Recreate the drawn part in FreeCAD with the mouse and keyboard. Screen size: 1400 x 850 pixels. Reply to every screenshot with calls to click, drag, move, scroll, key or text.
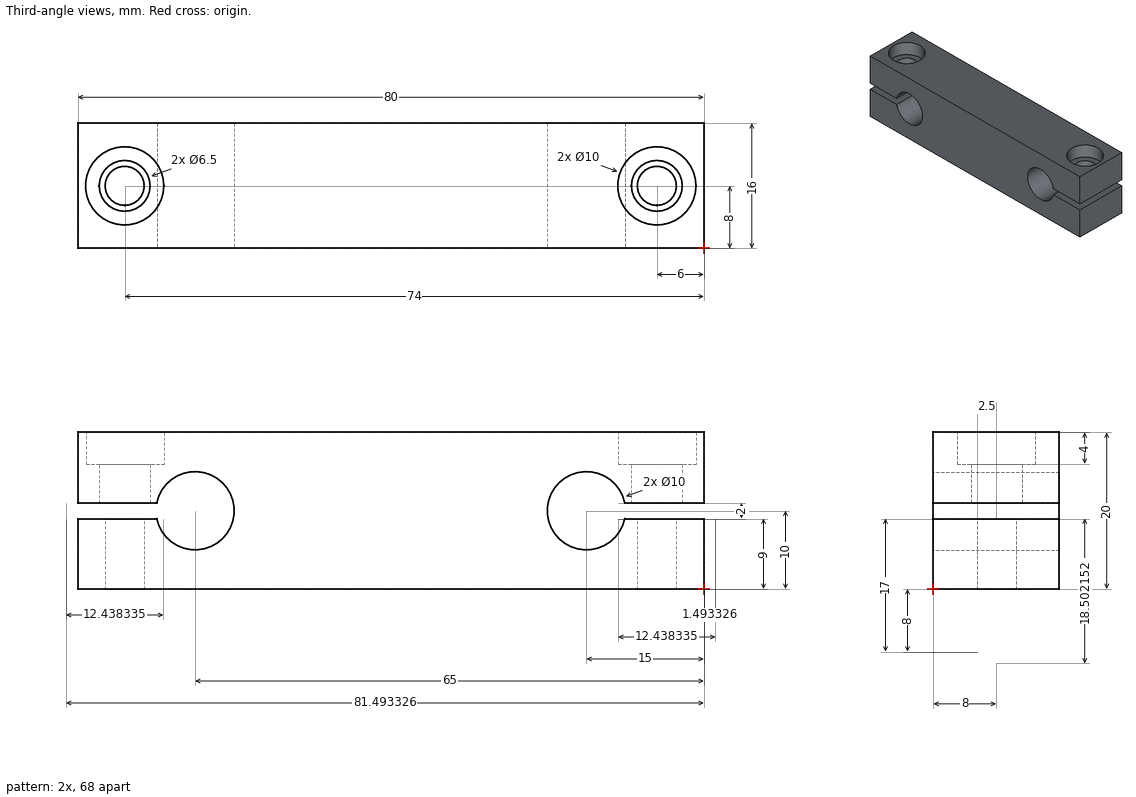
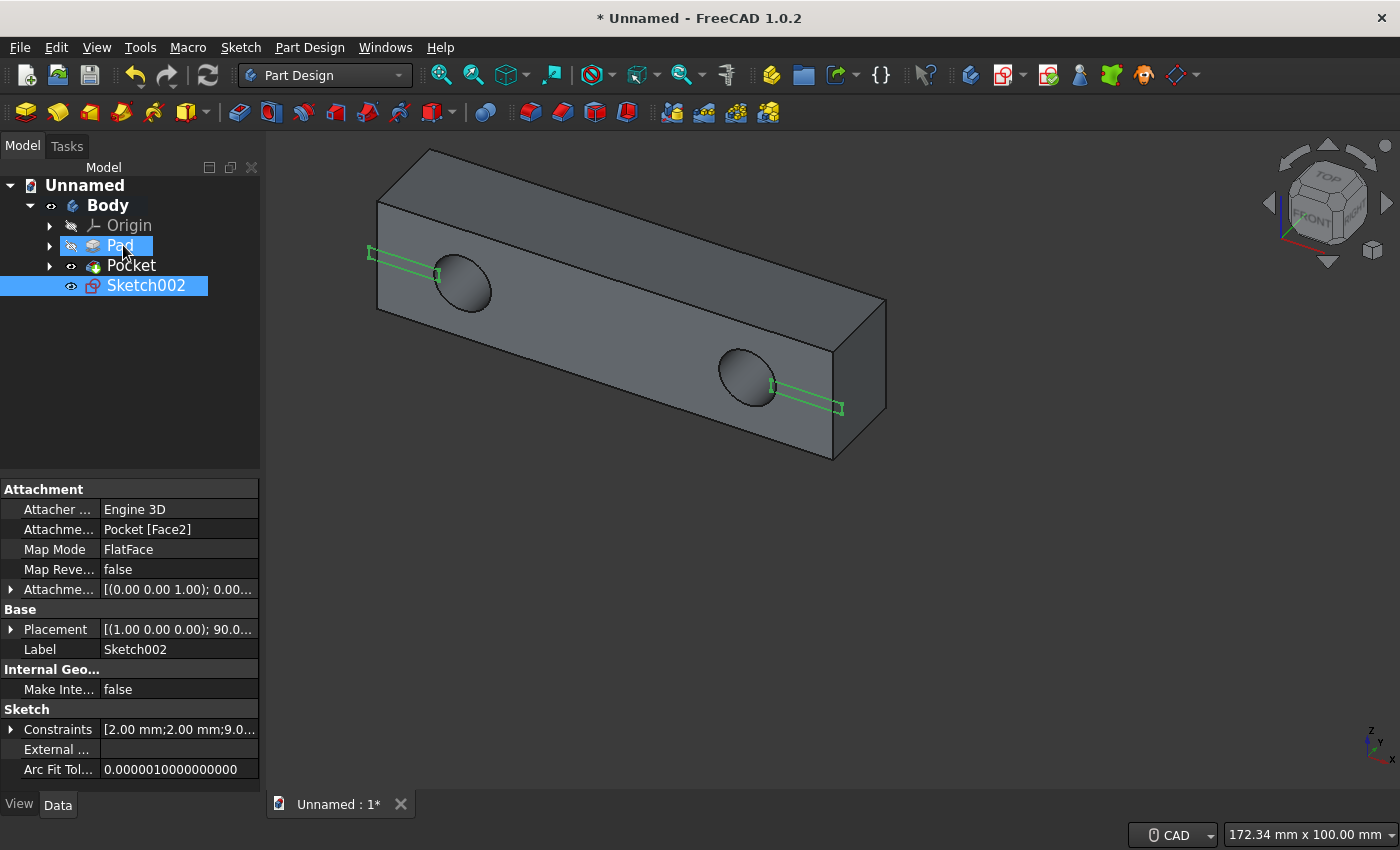
click(240, 112)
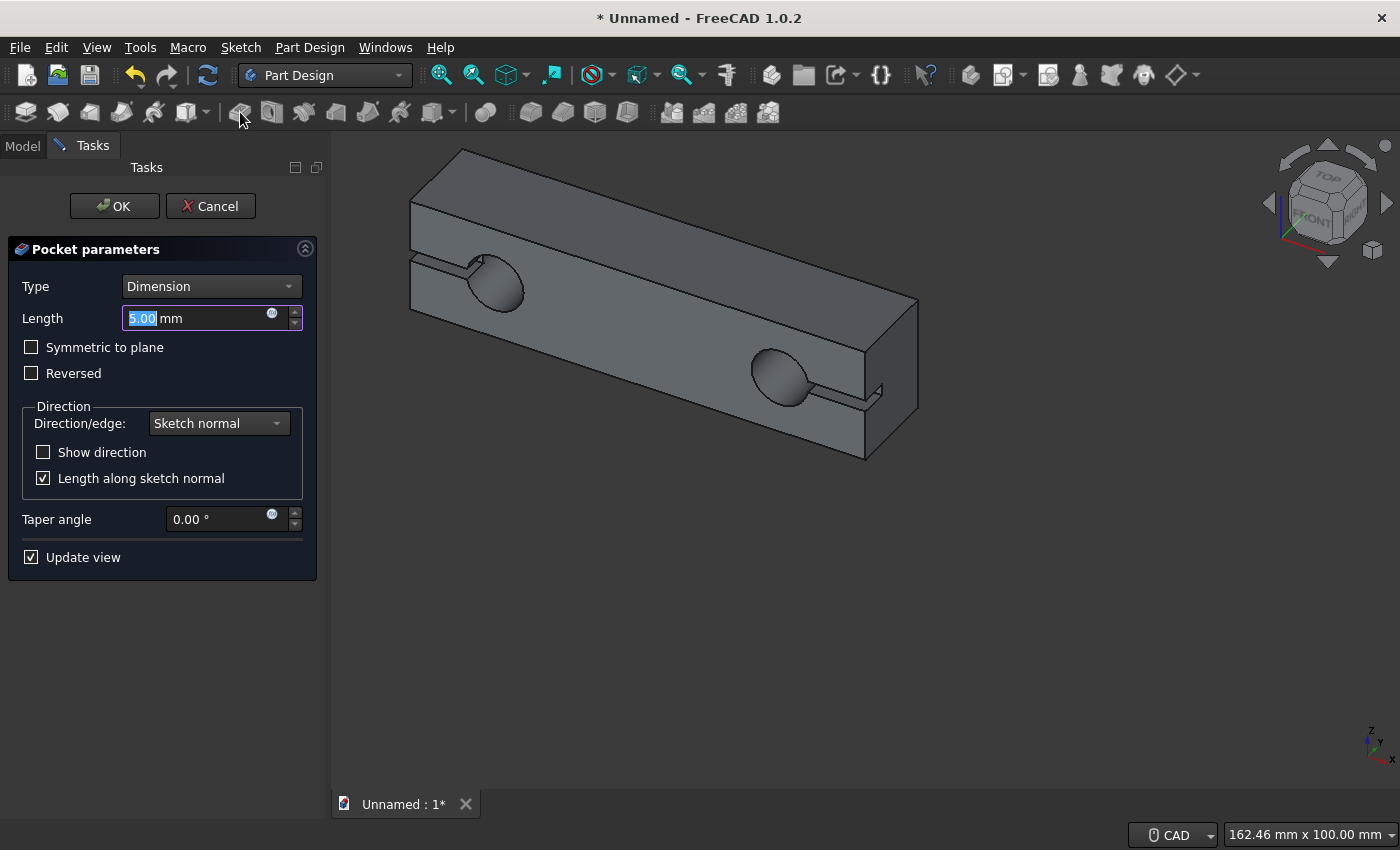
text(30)
key(Tab)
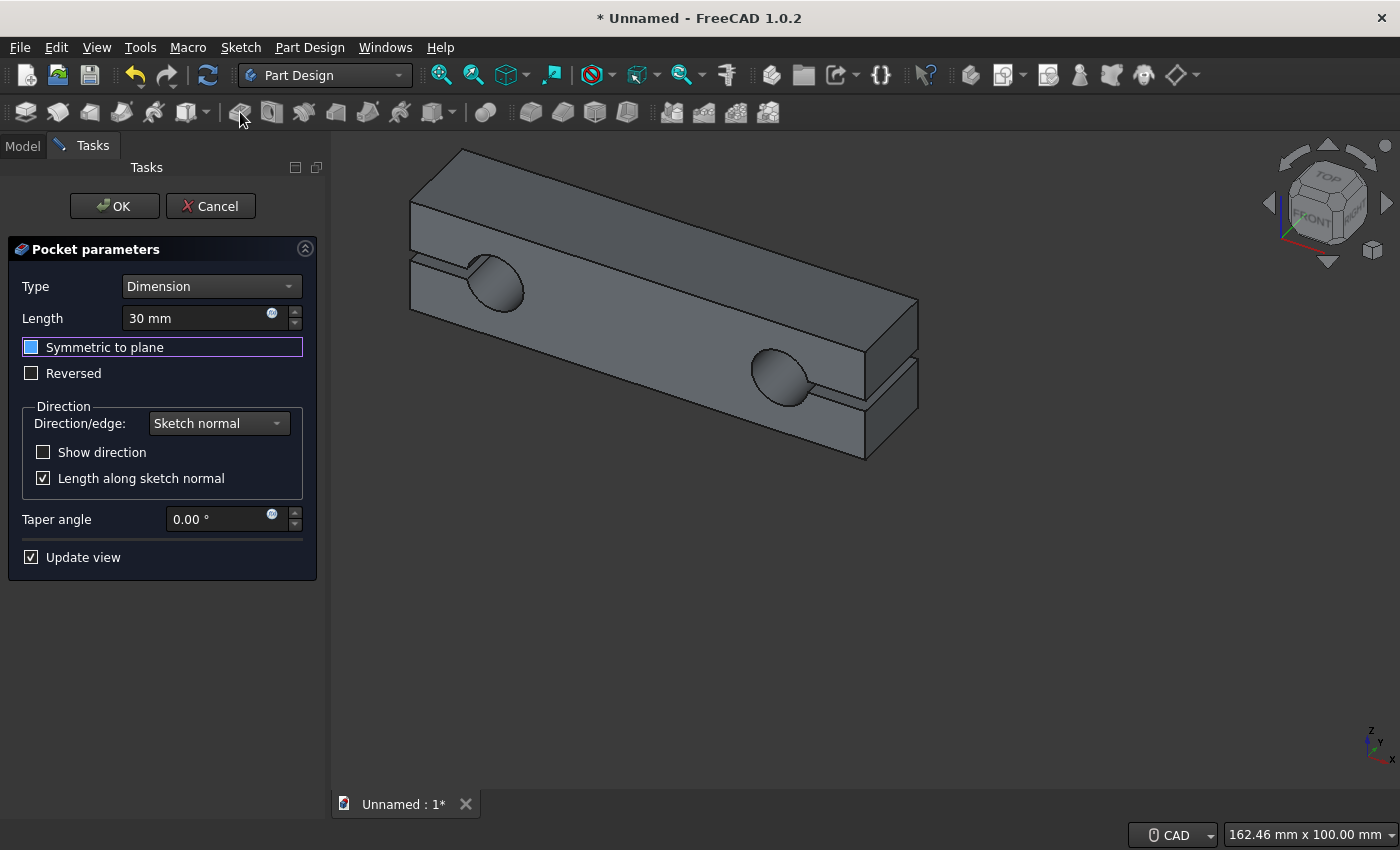
click(115, 206)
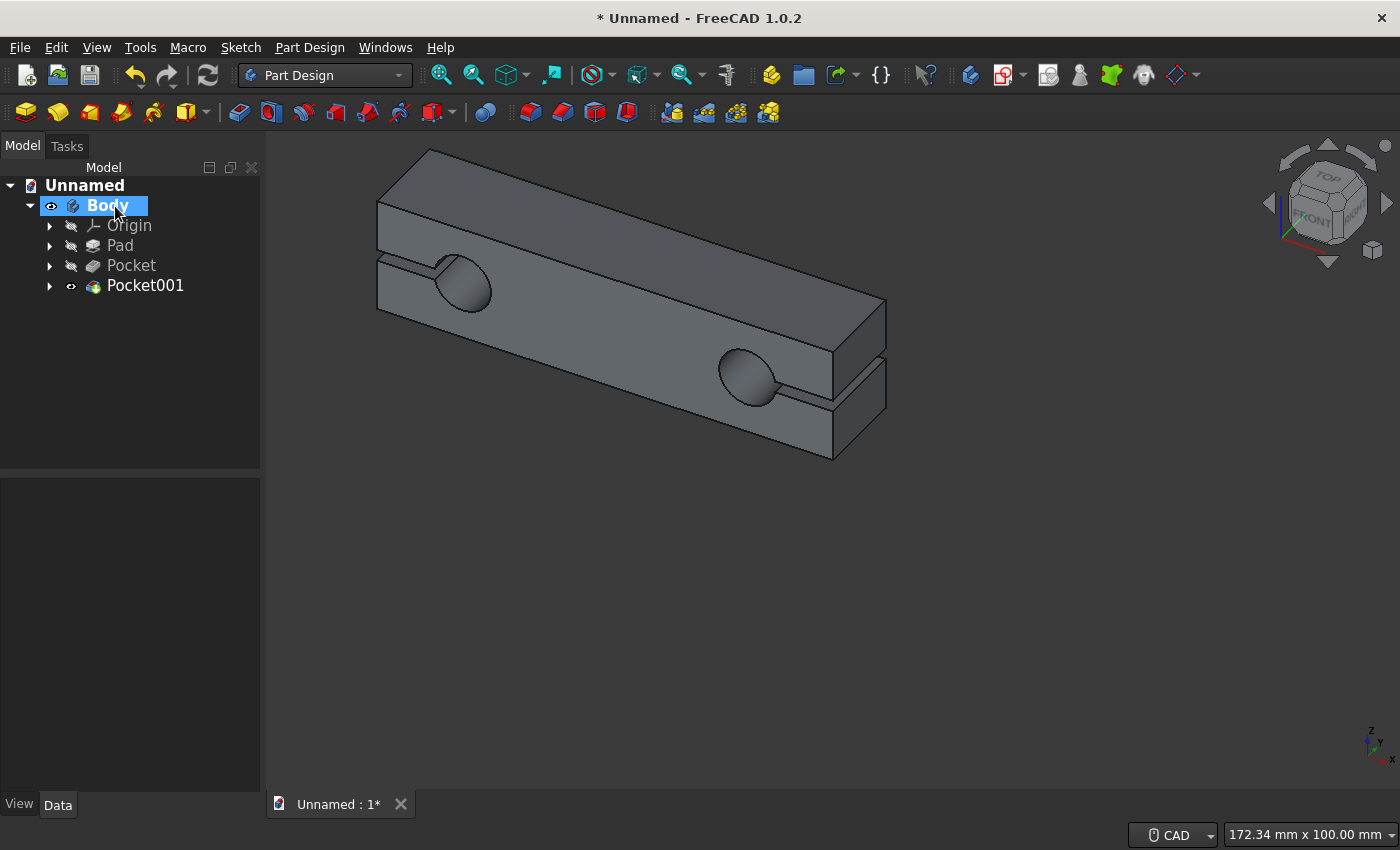
click(50, 226)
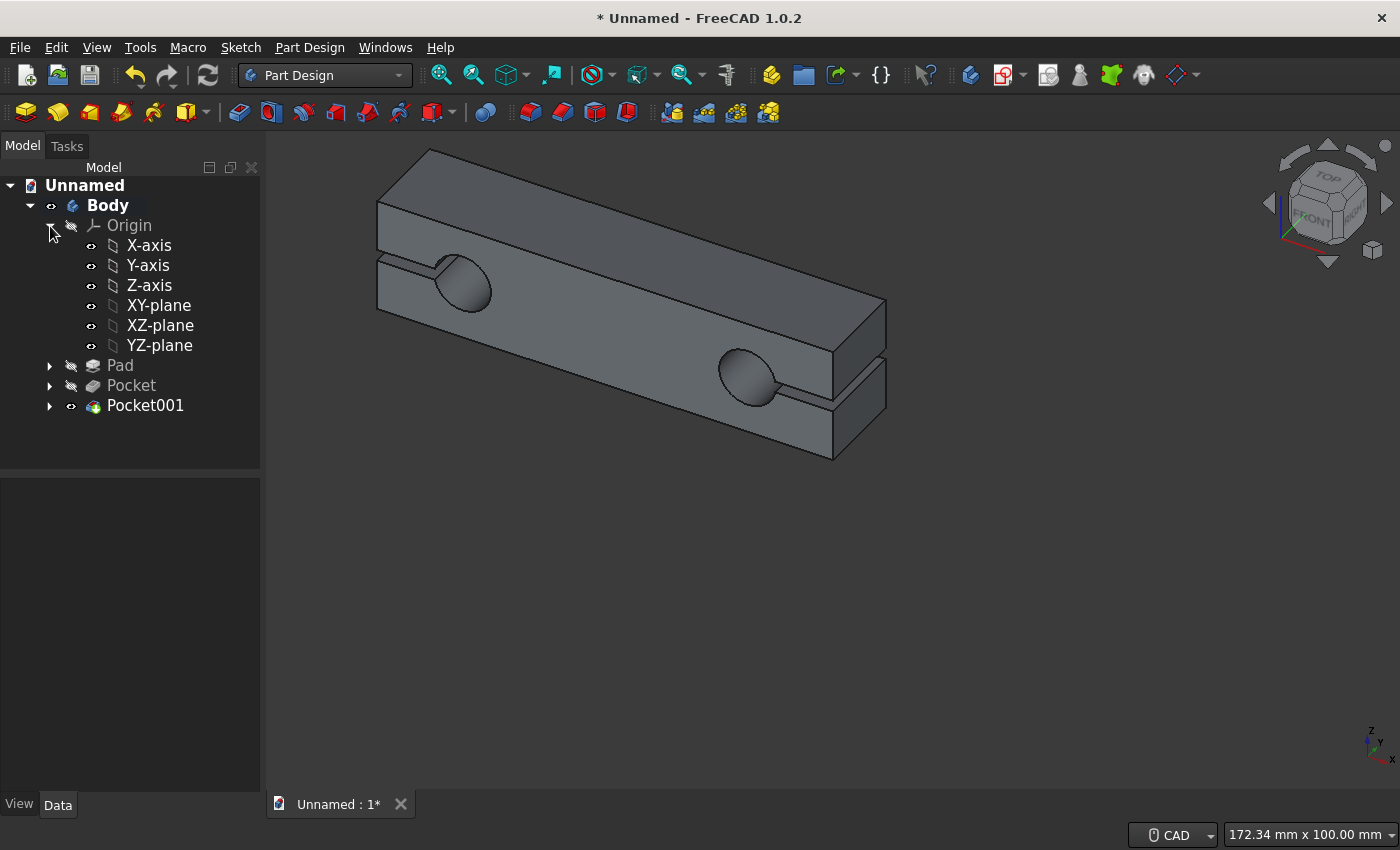
click(136, 346)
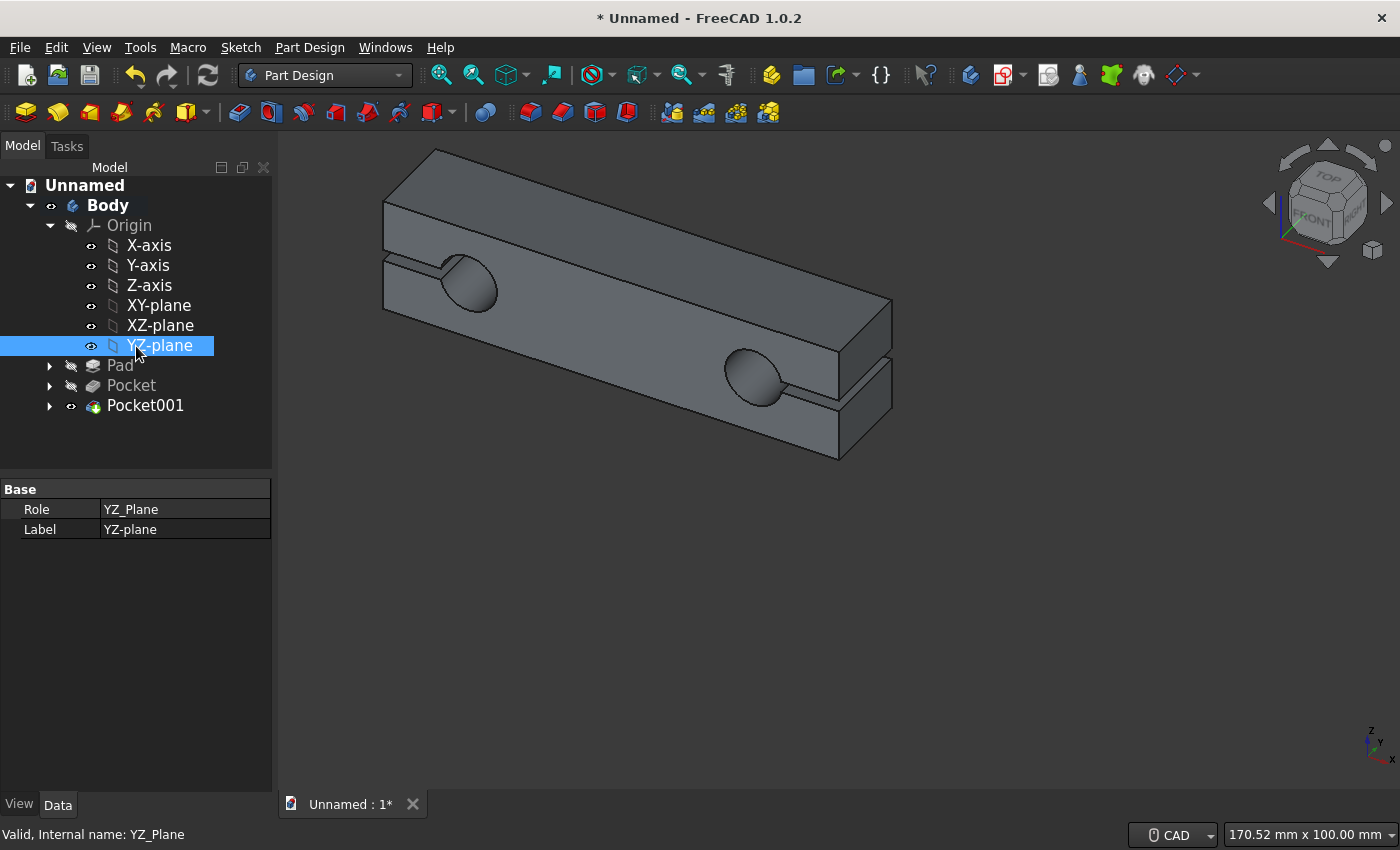
click(1176, 76)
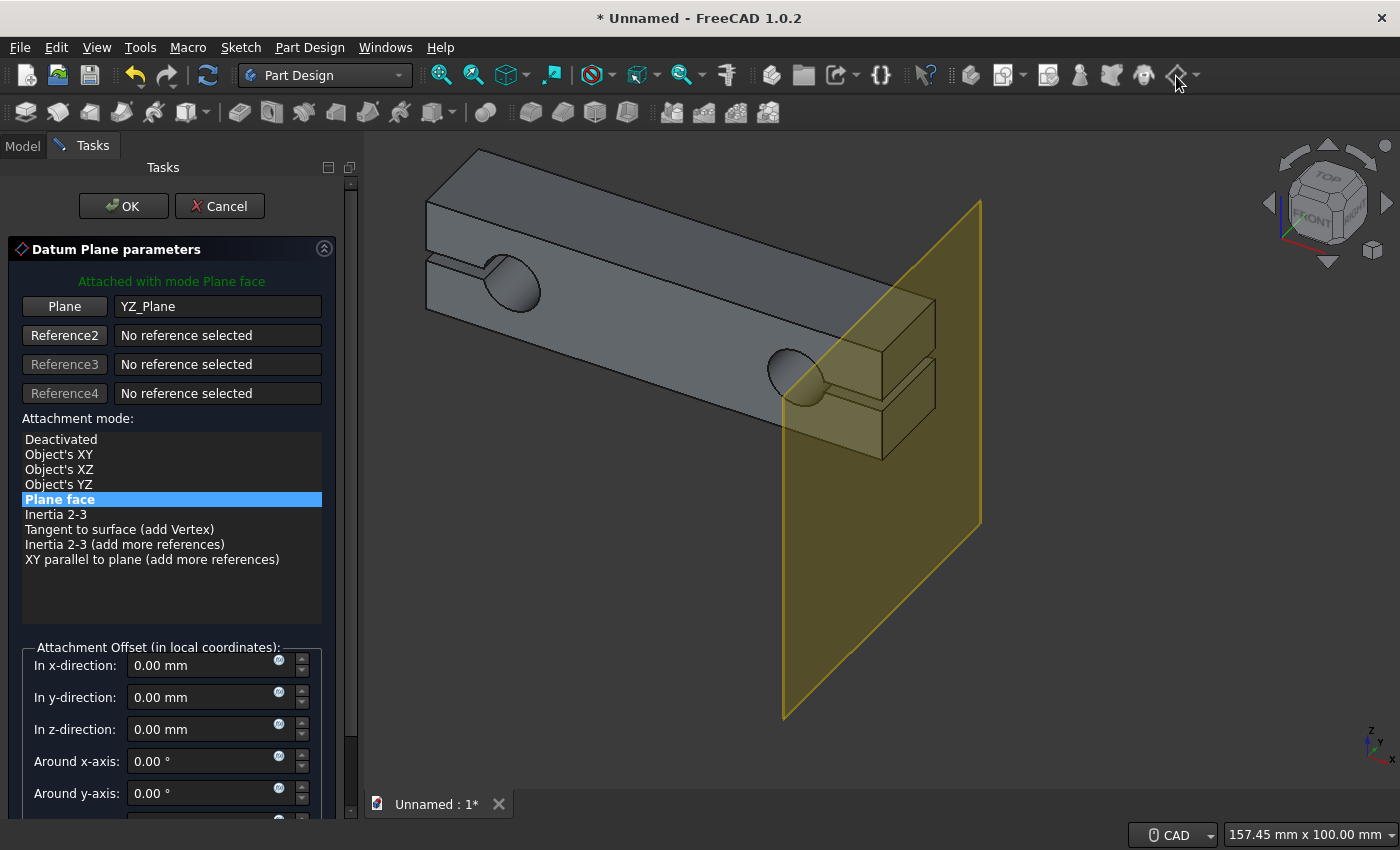
triple_click(210, 729)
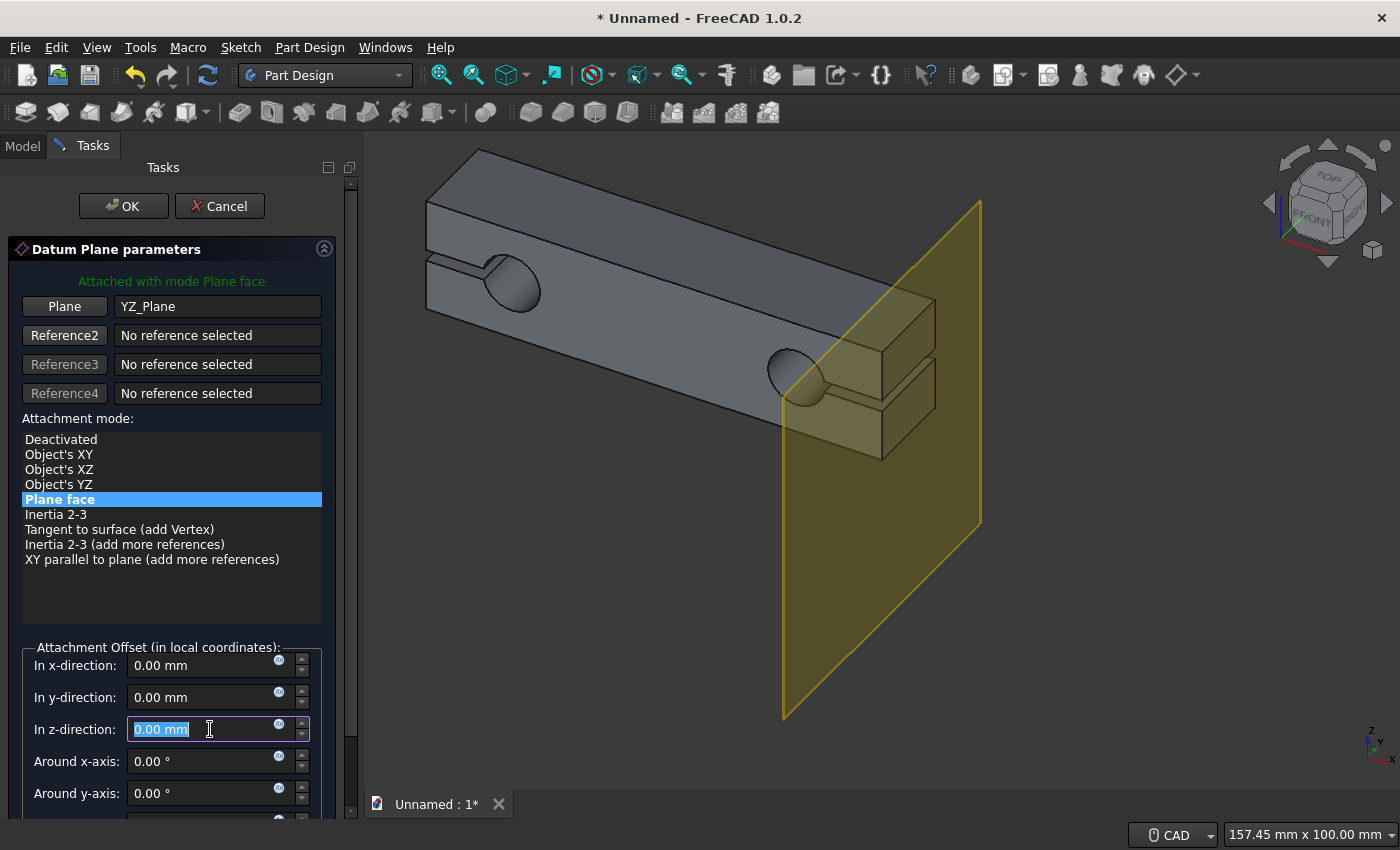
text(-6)
key(Tab)